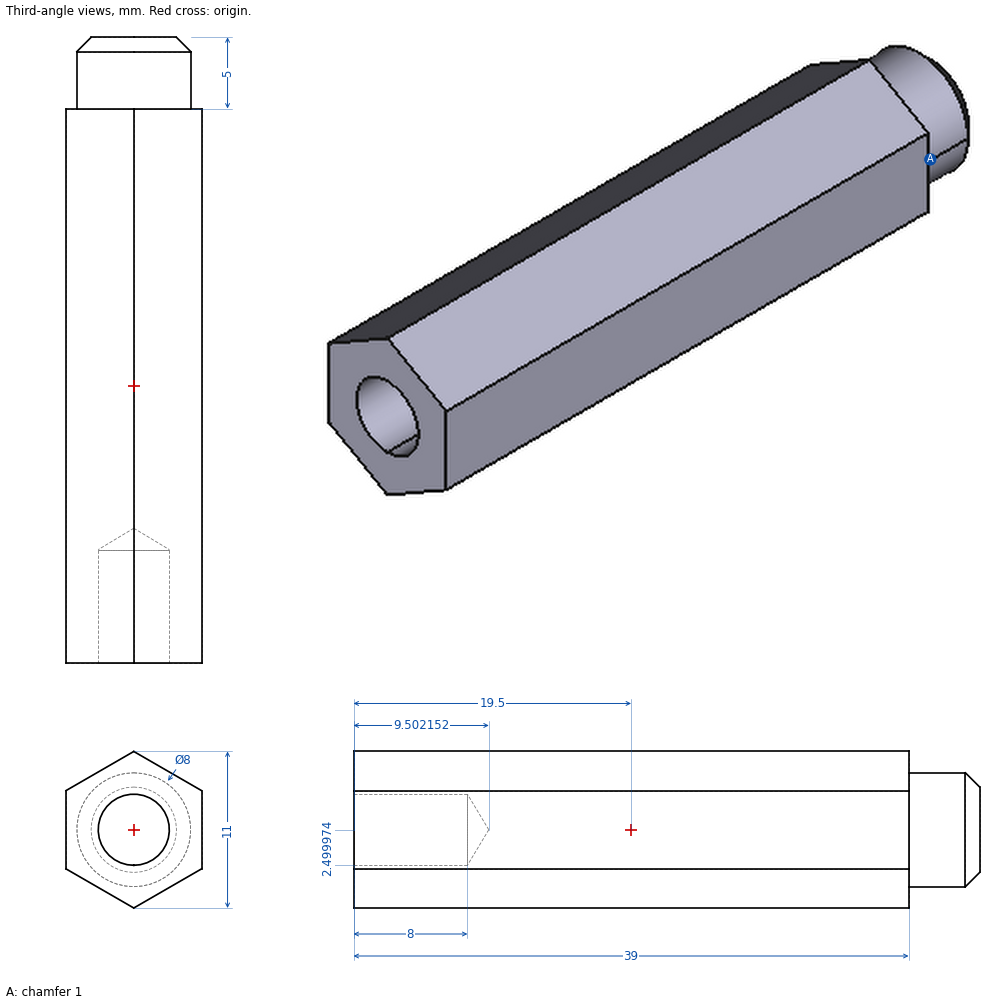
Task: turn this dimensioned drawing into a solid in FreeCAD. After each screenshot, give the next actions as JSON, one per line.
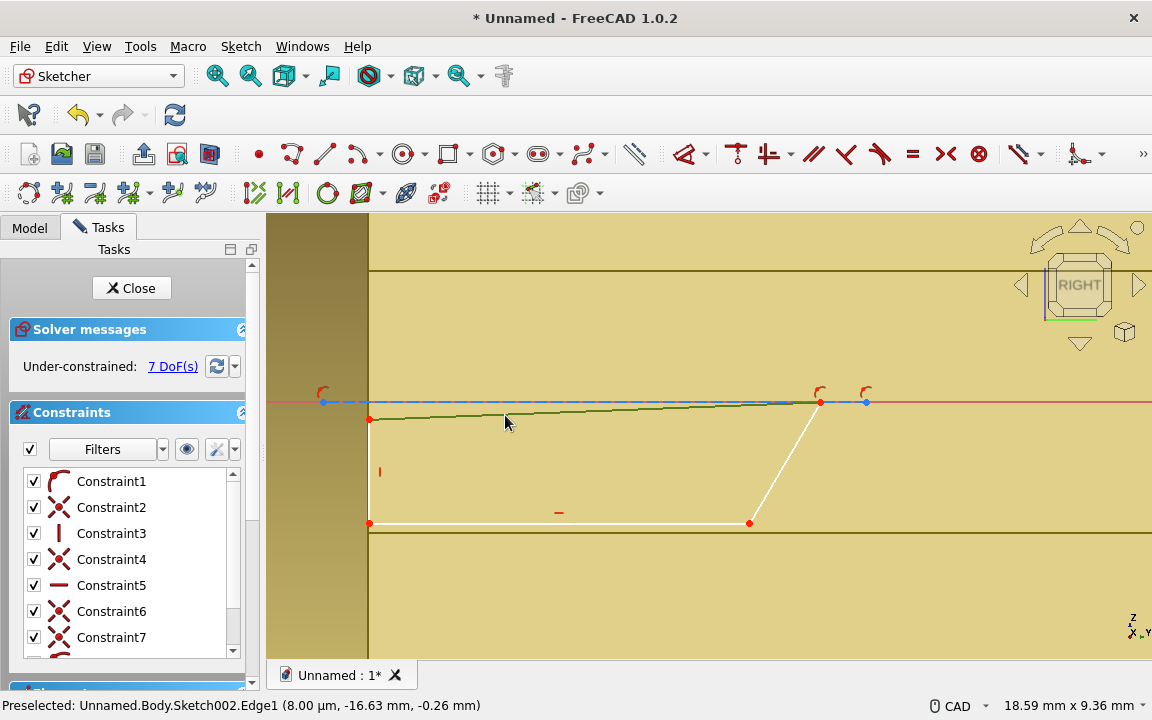
{"action": "key", "text": "h"}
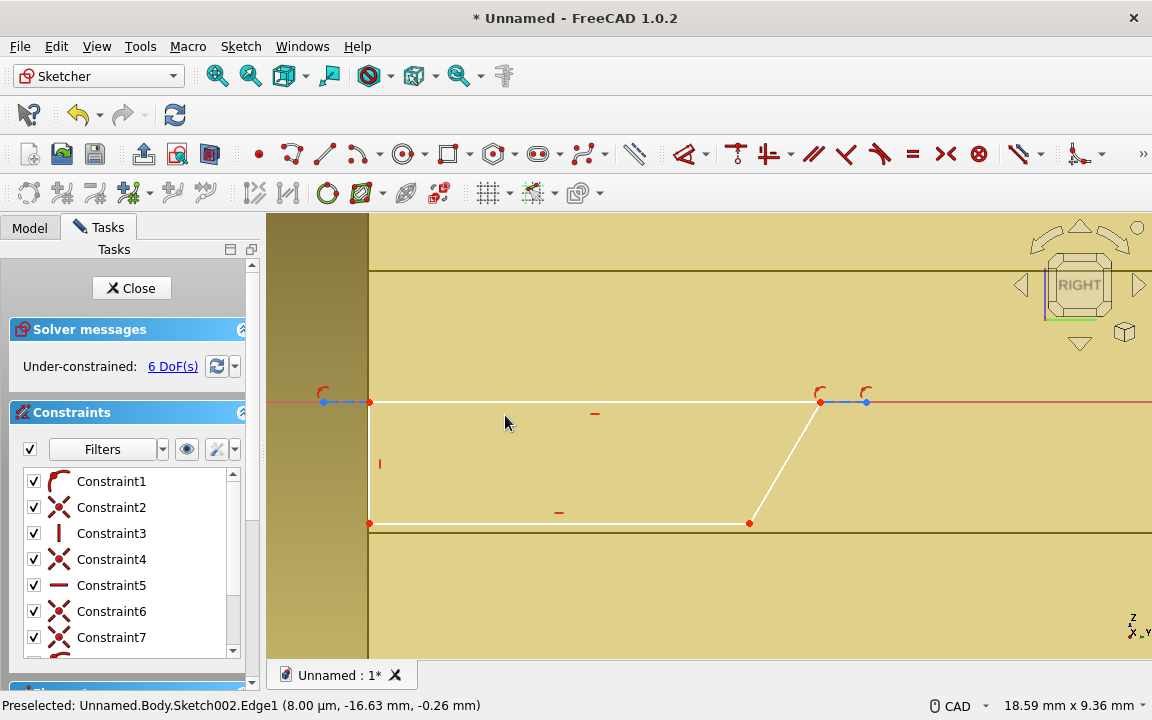
{"action": "key", "text": "d"}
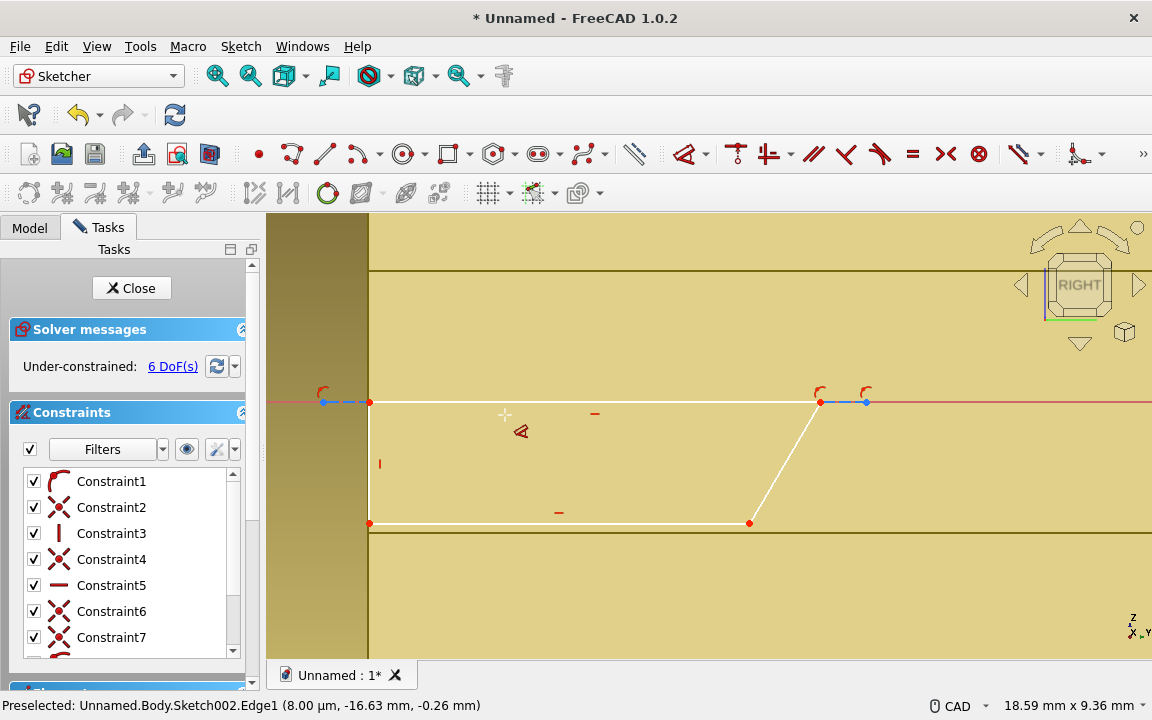
{"action": "left_click", "coordinate": [483, 524]}
{"action": "left_click", "coordinate": [559, 558]}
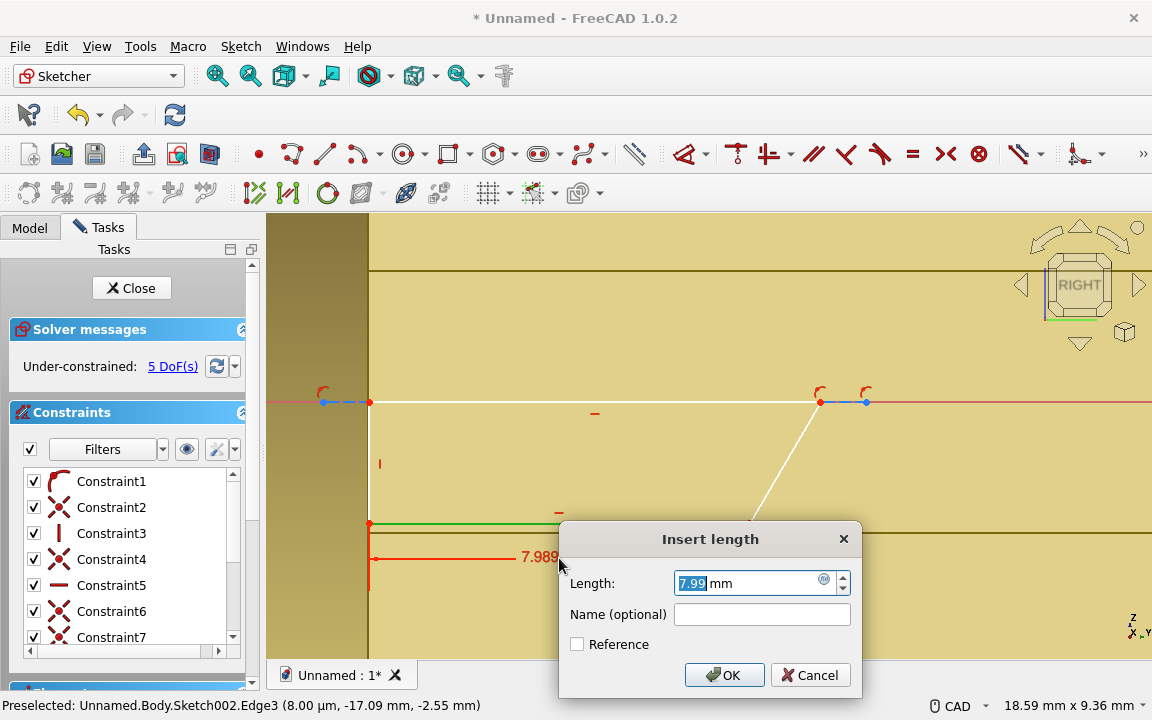
{"action": "type", "text": "8"}
{"action": "key", "text": "Return"}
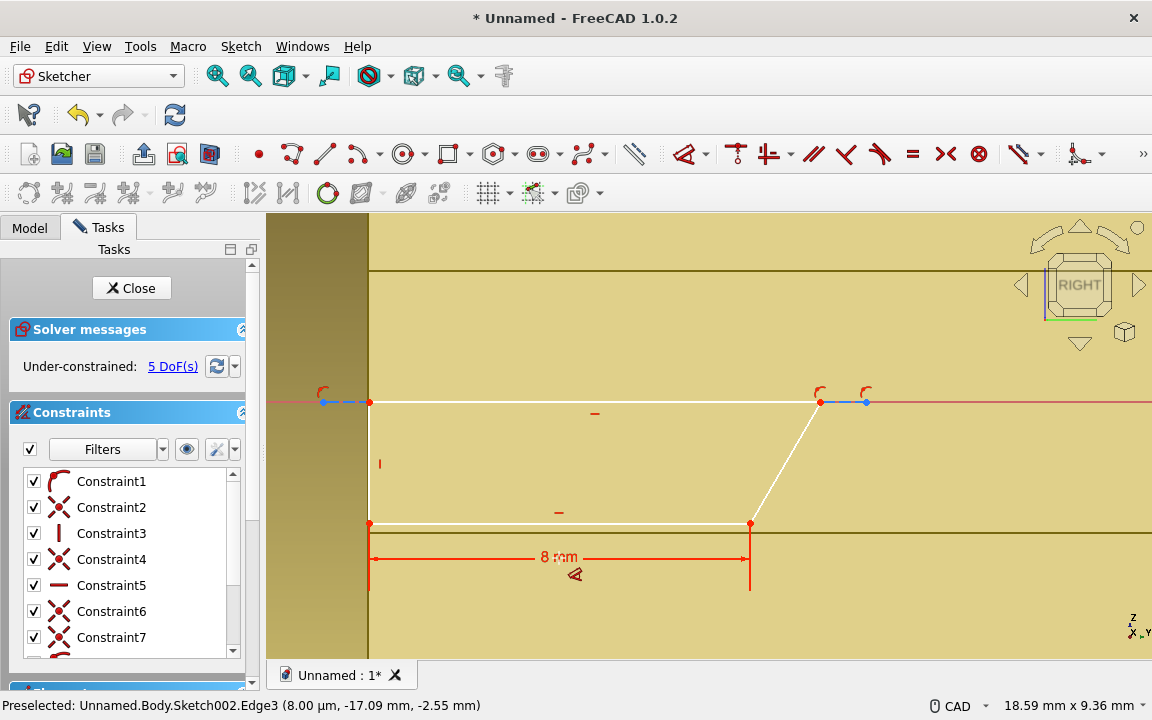
{"action": "left_click", "coordinate": [369, 402]}
{"action": "left_click", "coordinate": [678, 368]}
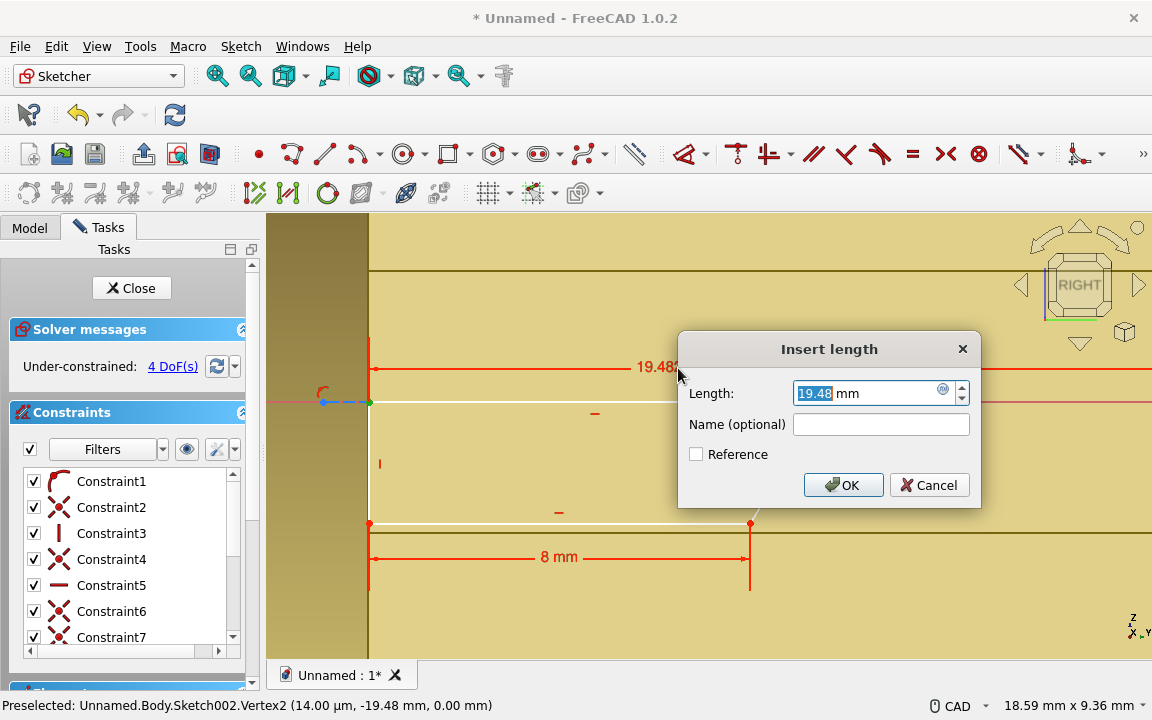
{"action": "type", "text": "19.5"}
{"action": "key", "text": "Return"}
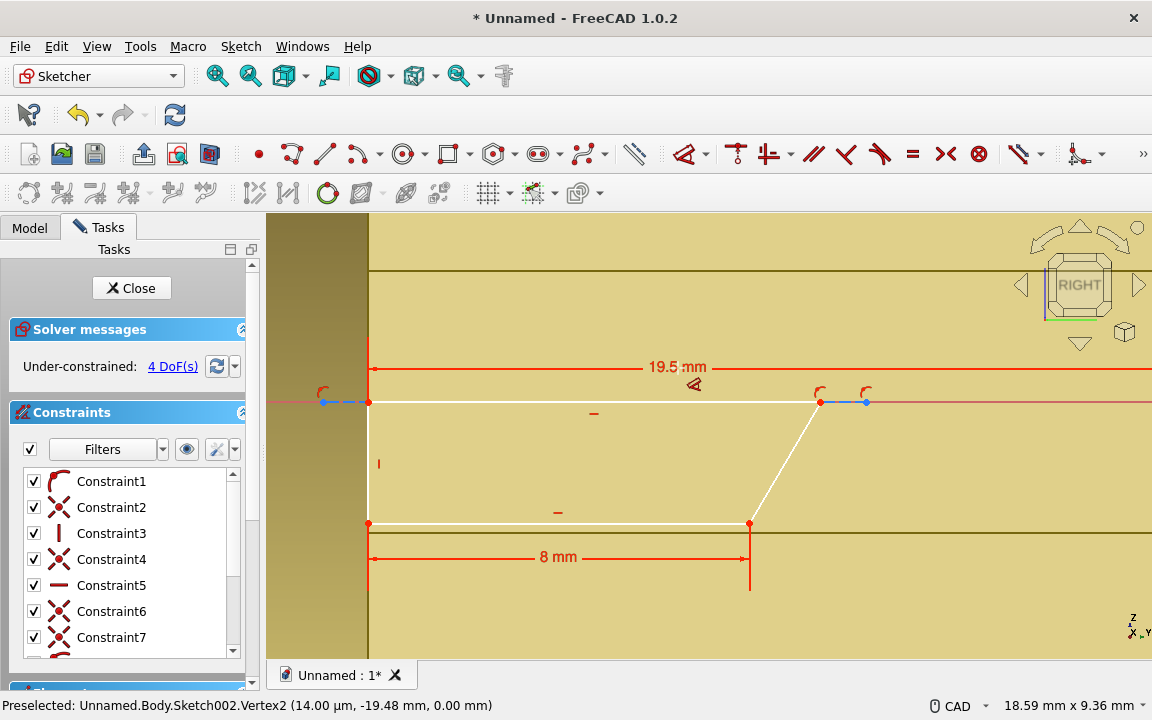
{"action": "scroll", "coordinate": [730, 402], "scroll_direction": "up", "scroll_amount": 11}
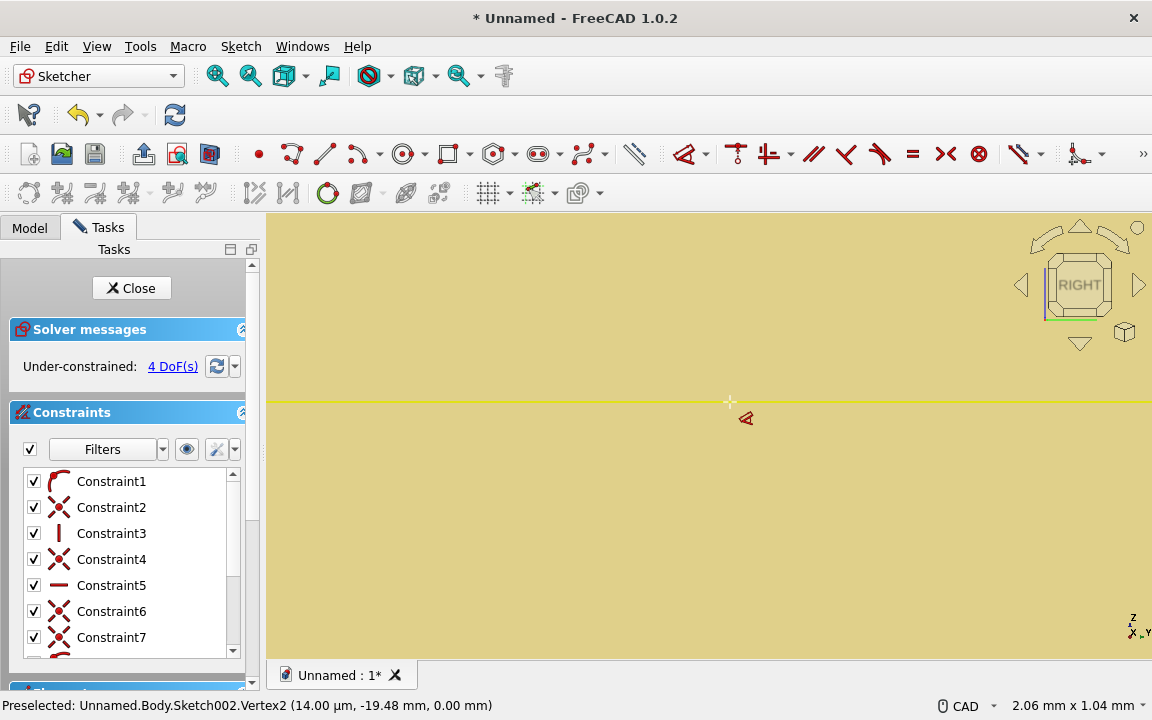
{"action": "left_click", "coordinate": [729, 402]}
{"action": "left_click", "coordinate": [640, 368]}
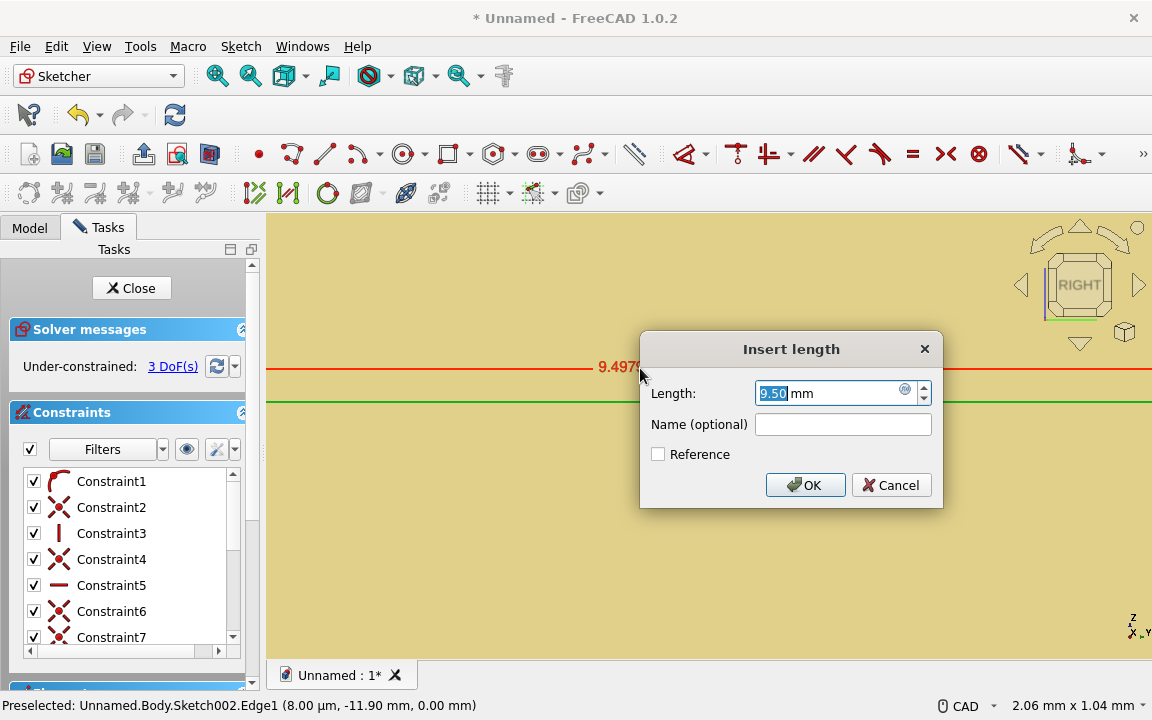
{"action": "type", "text": "9.502152"}
{"action": "key", "text": "Return"}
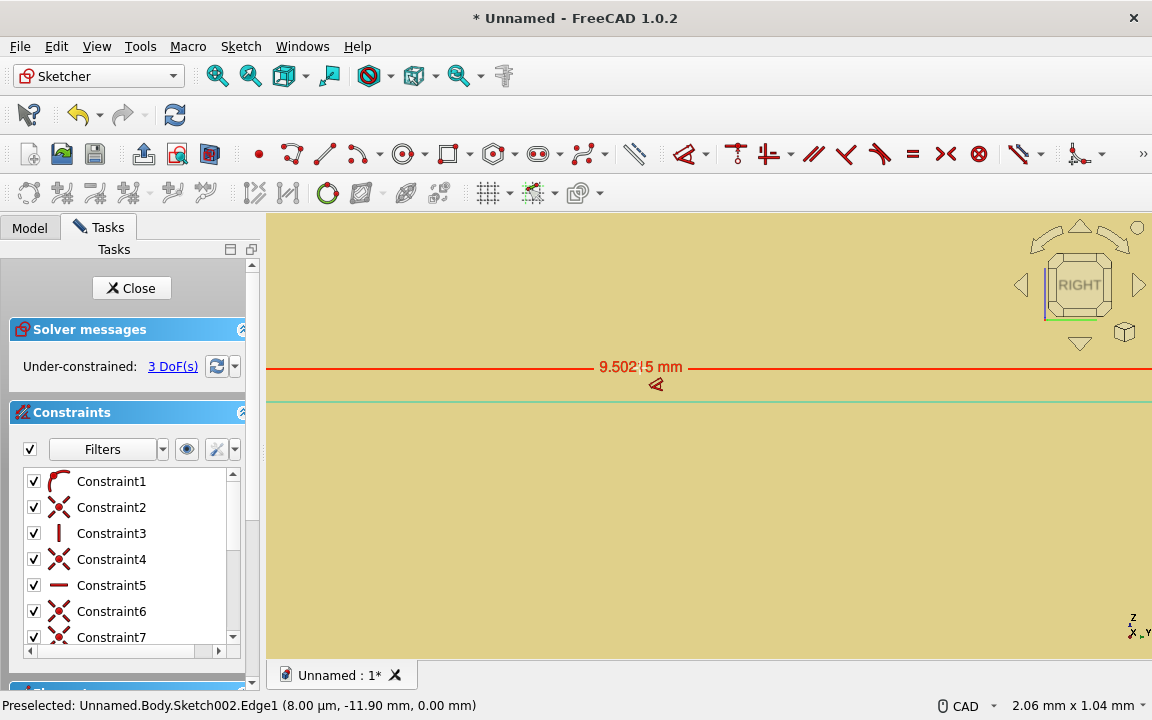
{"action": "scroll", "coordinate": [588, 403], "scroll_direction": "down", "scroll_amount": 14}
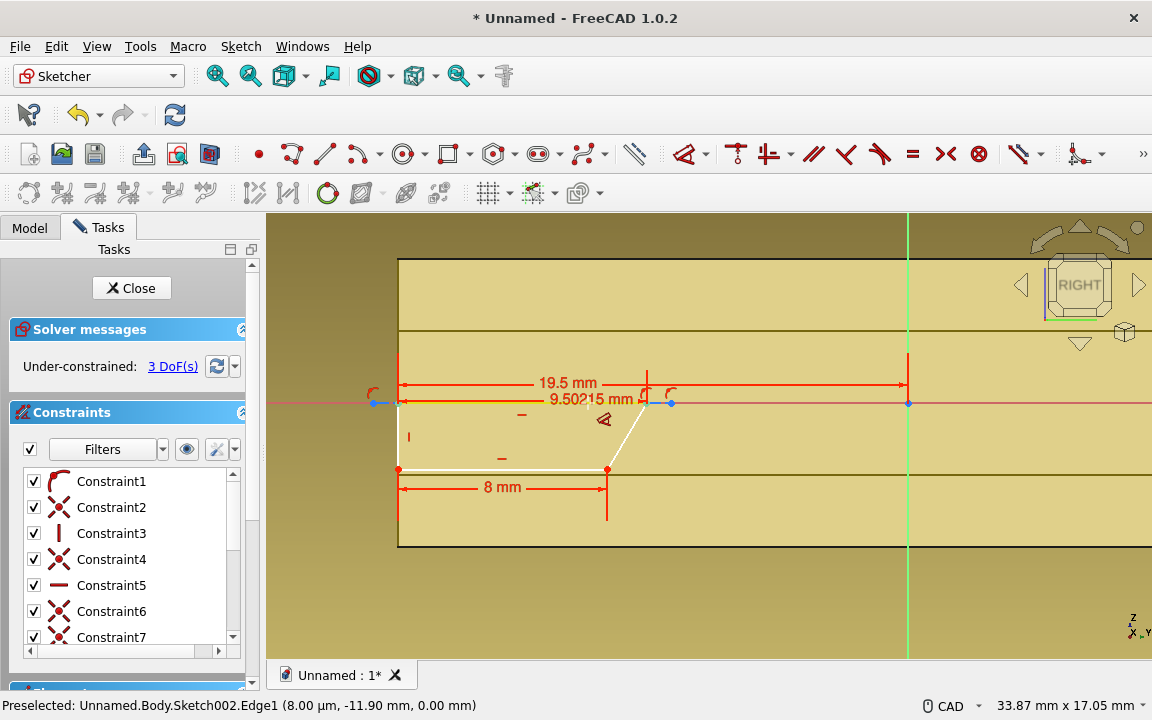
{"action": "left_click", "coordinate": [398, 423]}
{"action": "left_click", "coordinate": [364, 437]}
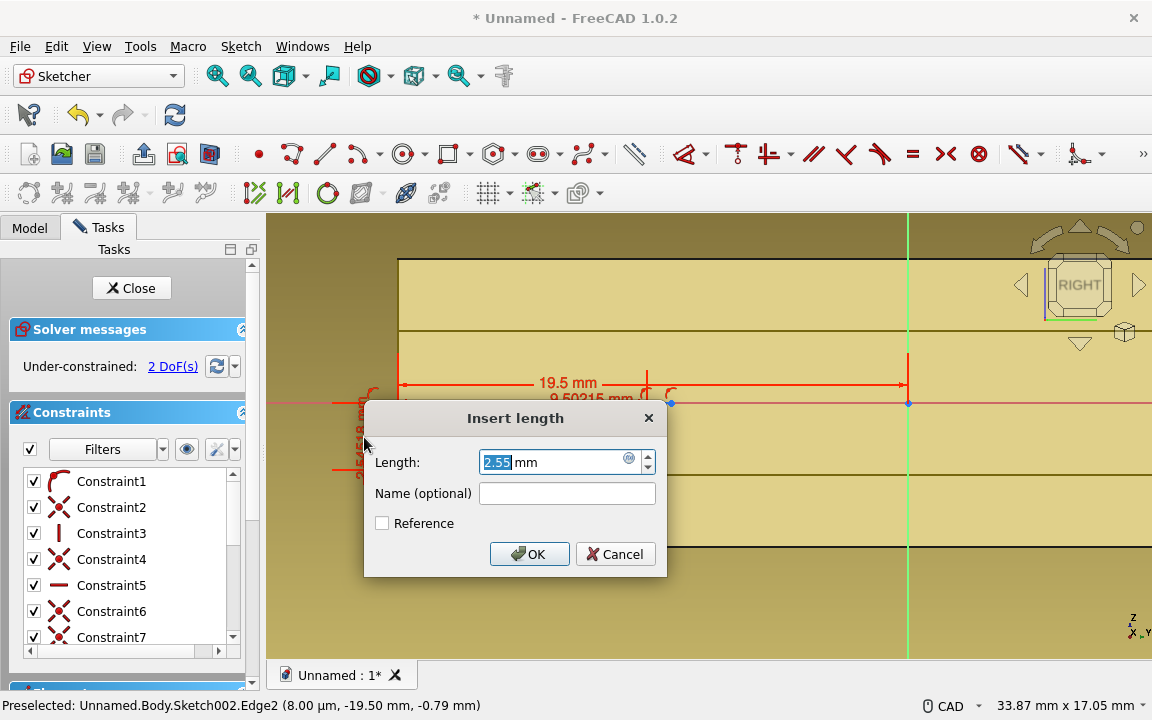
{"action": "type", "text": "2.499974"}
{"action": "key", "text": "Return"}
{"action": "key", "text": "Escape"}